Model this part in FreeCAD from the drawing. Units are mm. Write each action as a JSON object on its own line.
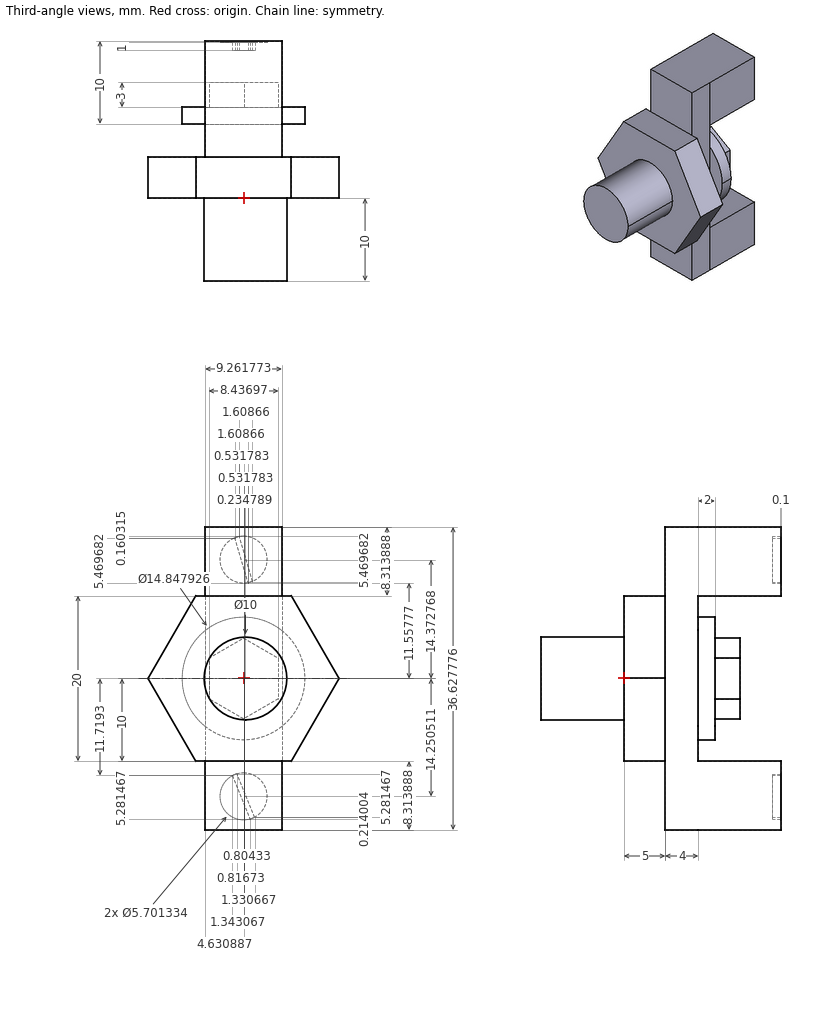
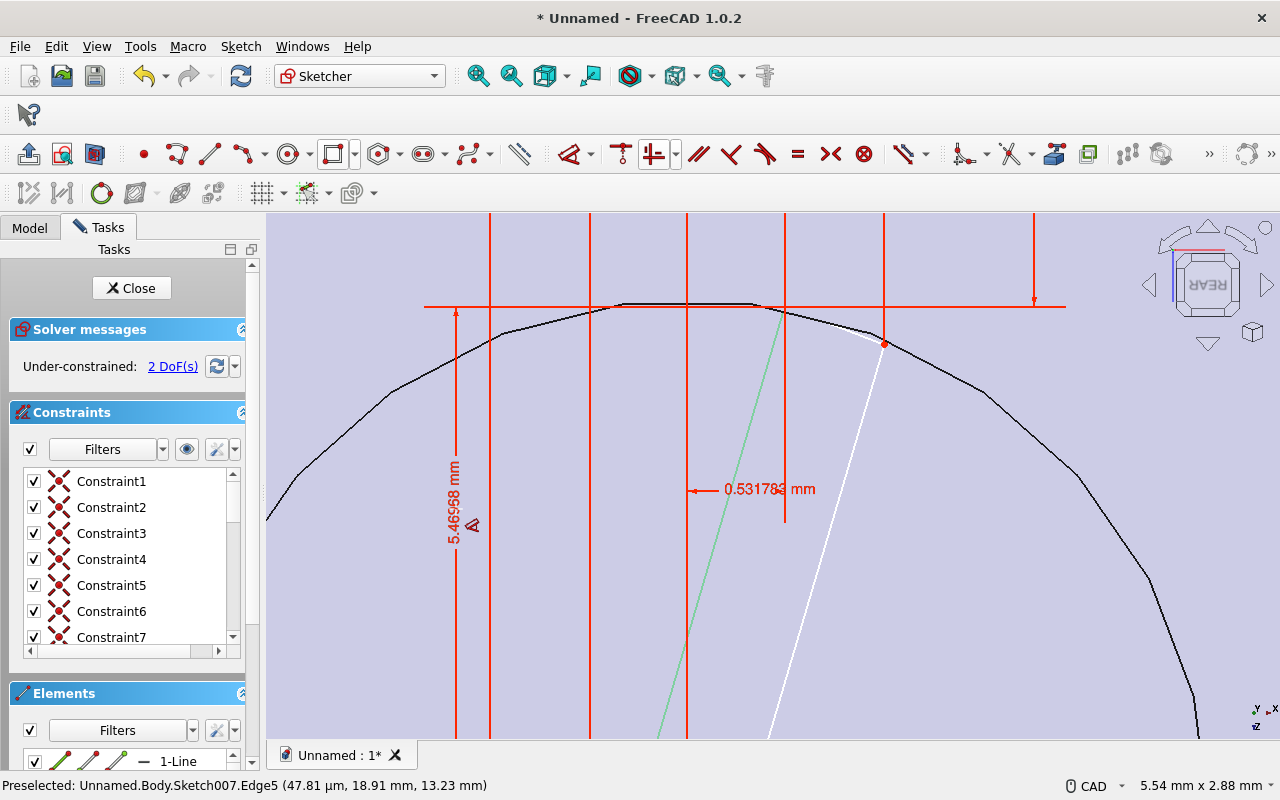
{"action": "scroll", "coordinate": [705, 595], "scroll_direction": "down", "scroll_amount": 15}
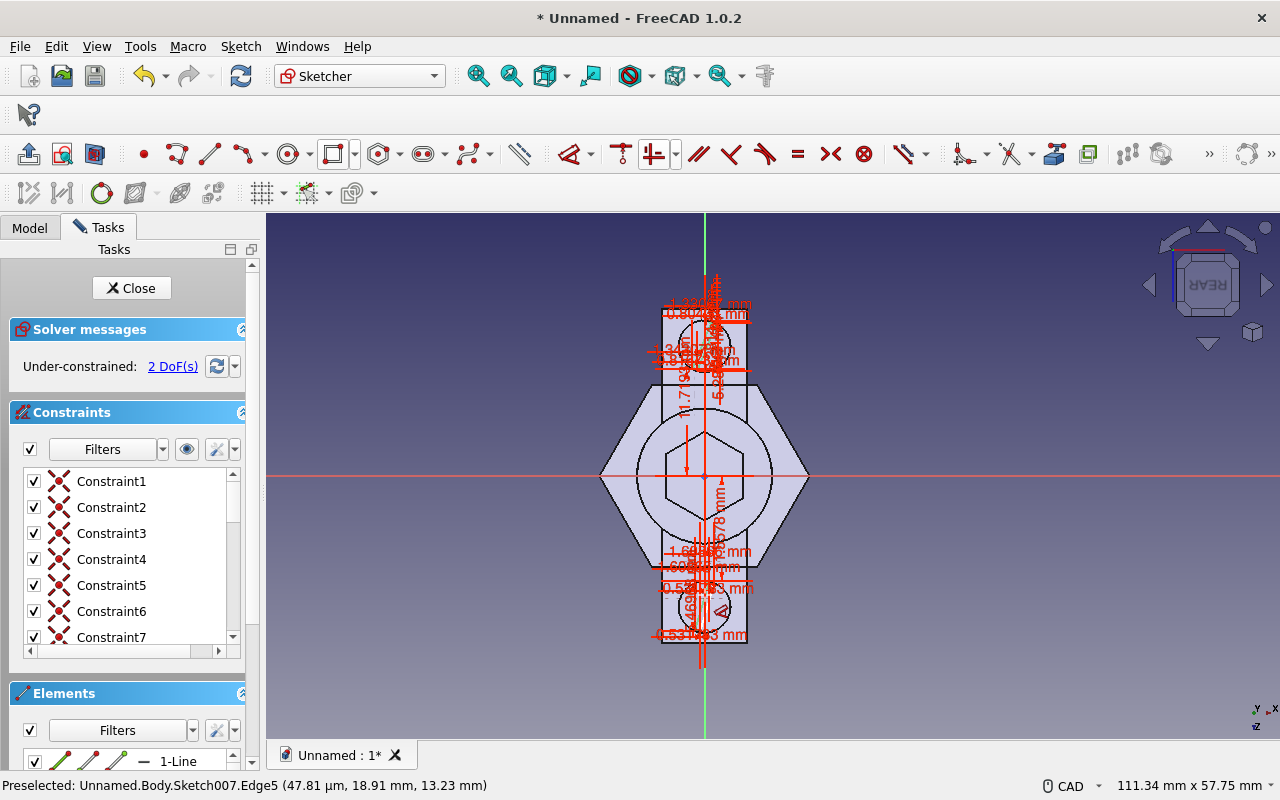
{"action": "scroll", "coordinate": [696, 632], "scroll_direction": "up", "scroll_amount": 17}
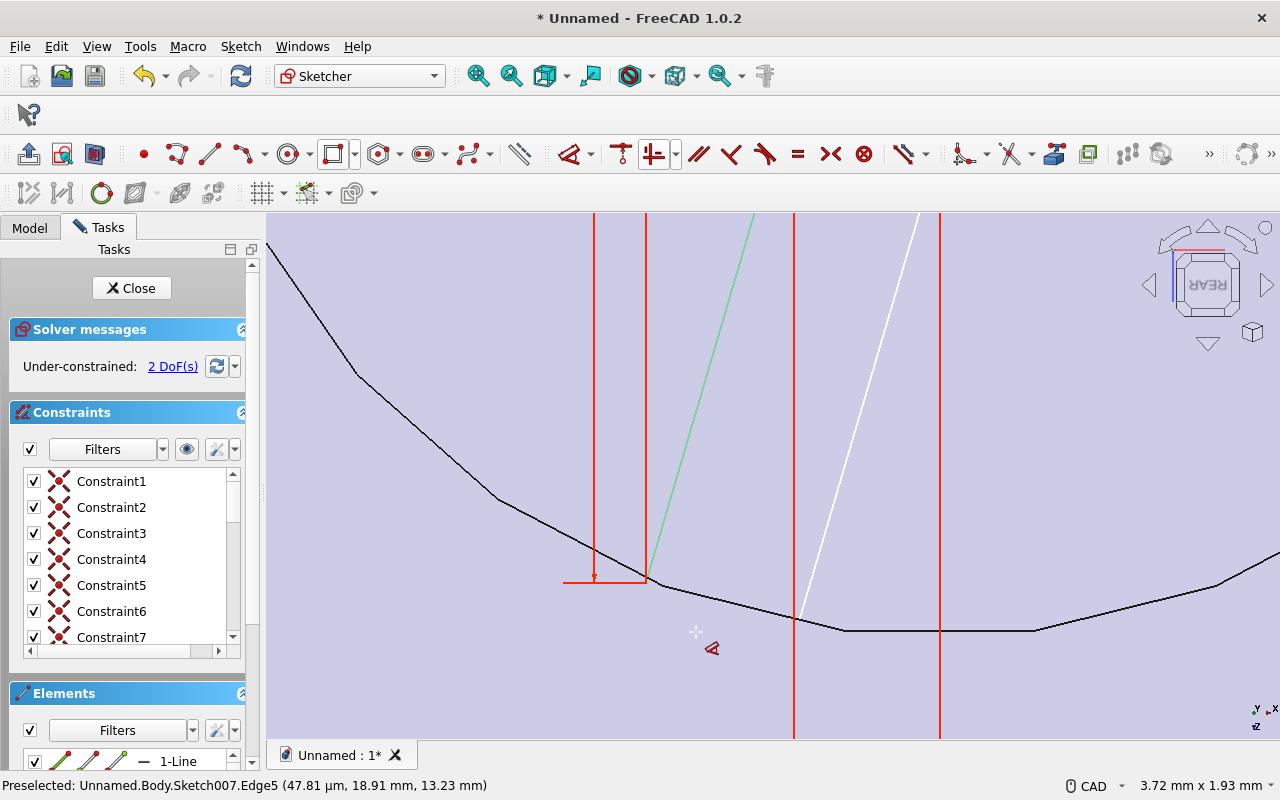
{"action": "left_click", "coordinate": [690, 599]}
{"action": "left_click", "coordinate": [612, 610]}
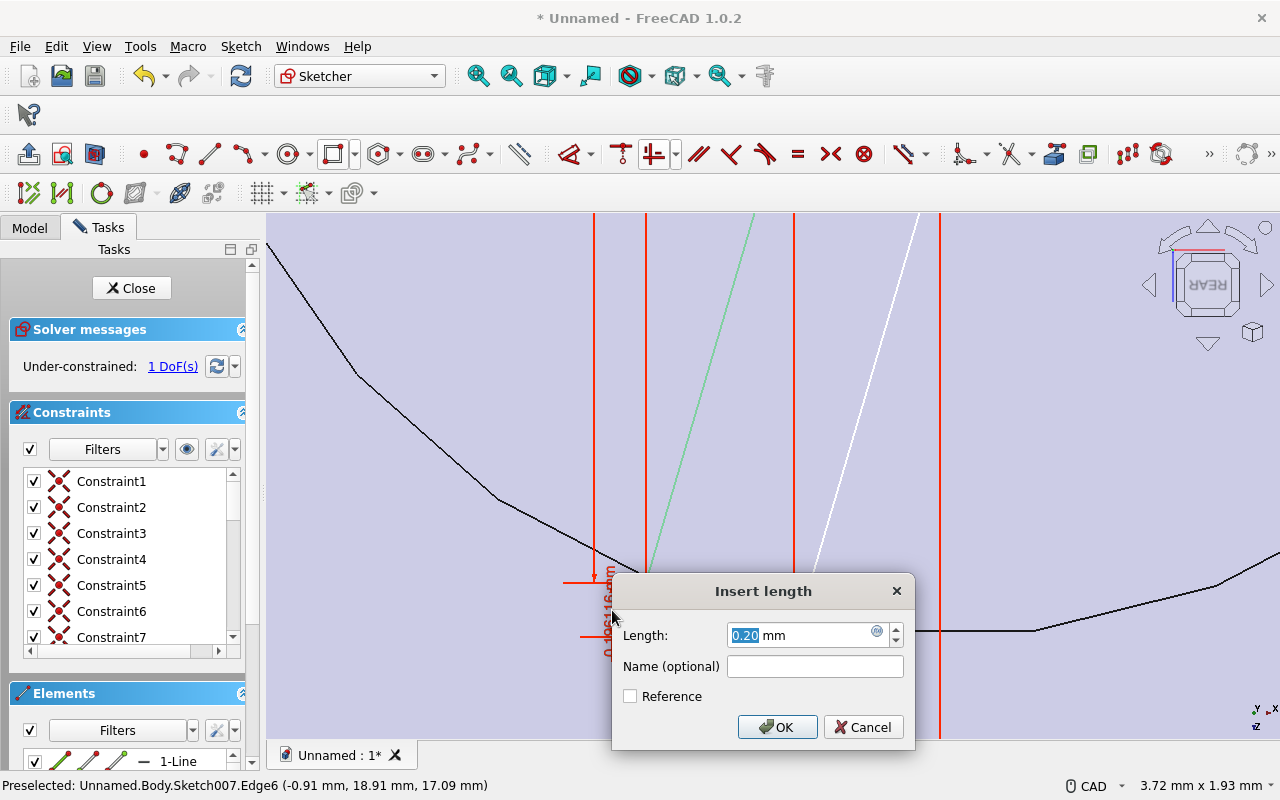
{"action": "type", "text": "0.160315"}
{"action": "key", "text": "Return"}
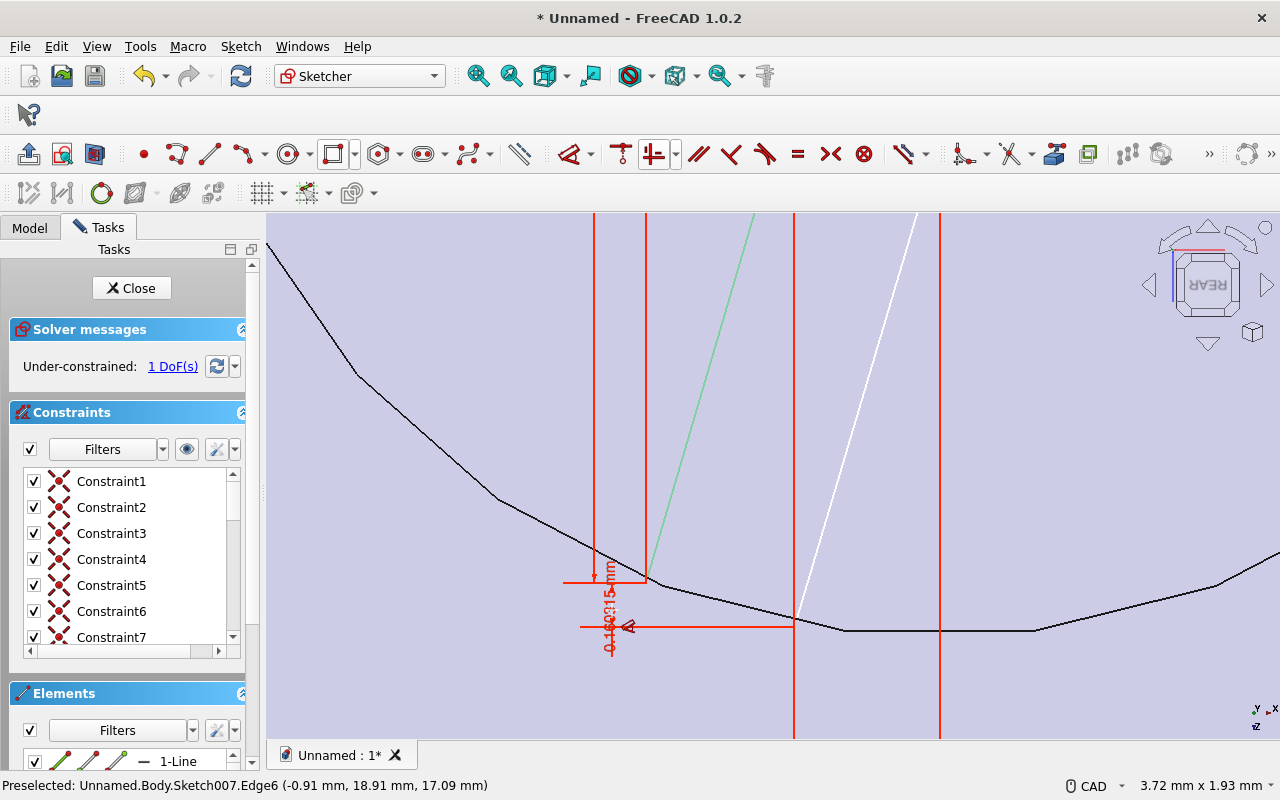
{"action": "scroll", "coordinate": [695, 668], "scroll_direction": "down", "scroll_amount": 16}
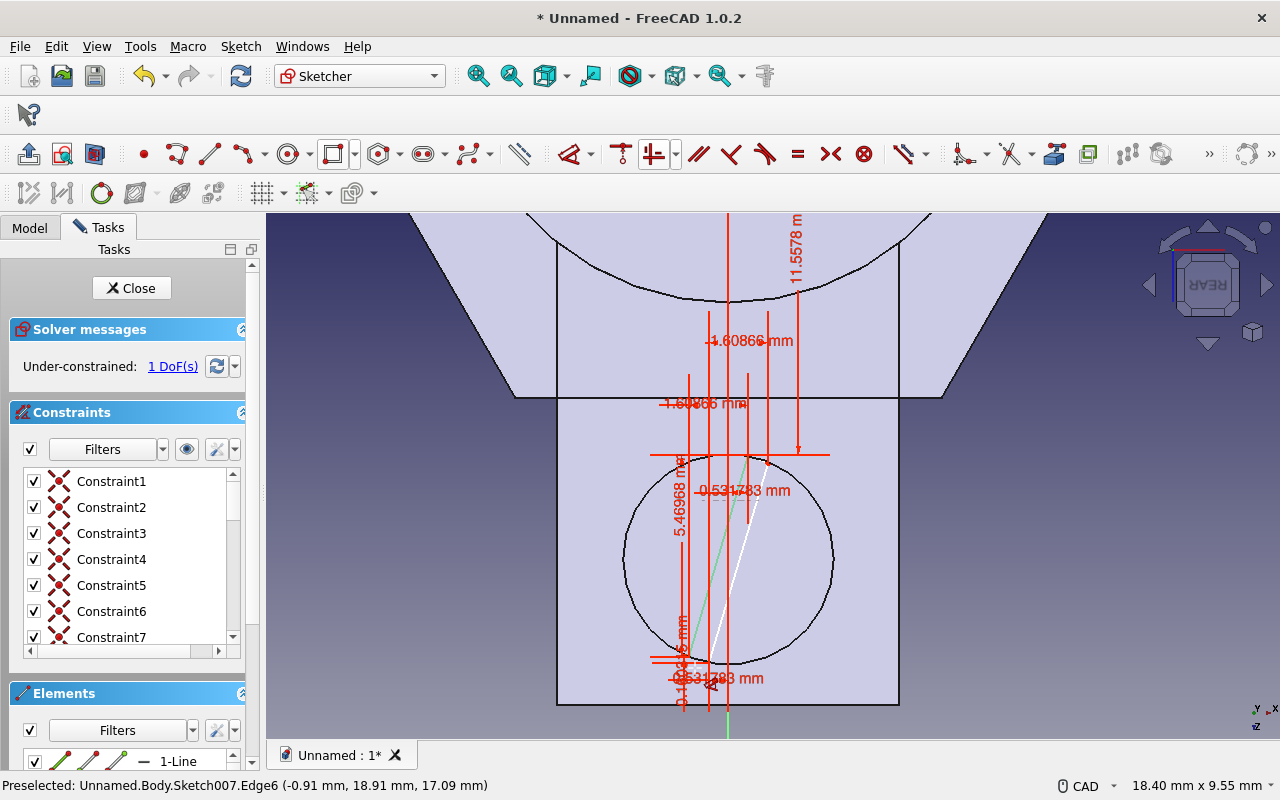
{"action": "scroll", "coordinate": [703, 655], "scroll_direction": "up", "scroll_amount": 9}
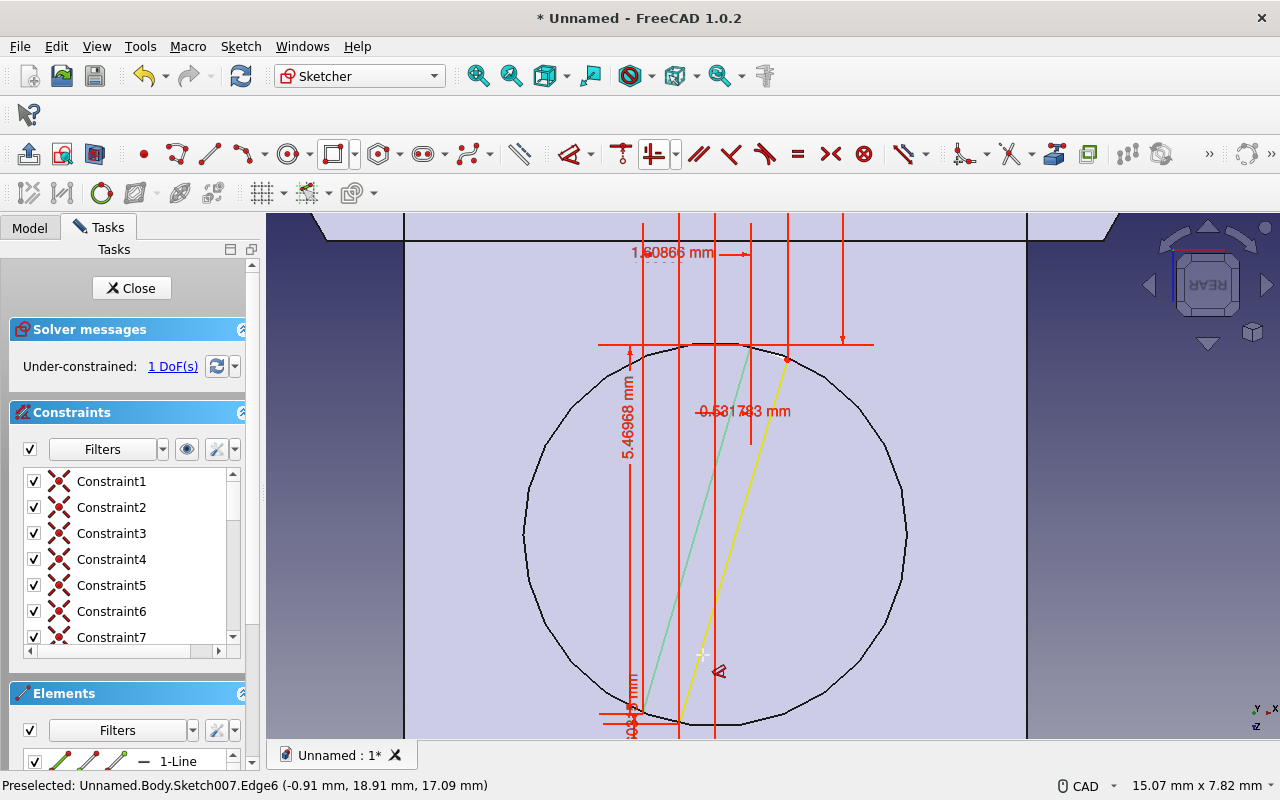
{"action": "left_click", "coordinate": [701, 651]}
{"action": "left_click", "coordinate": [822, 535]}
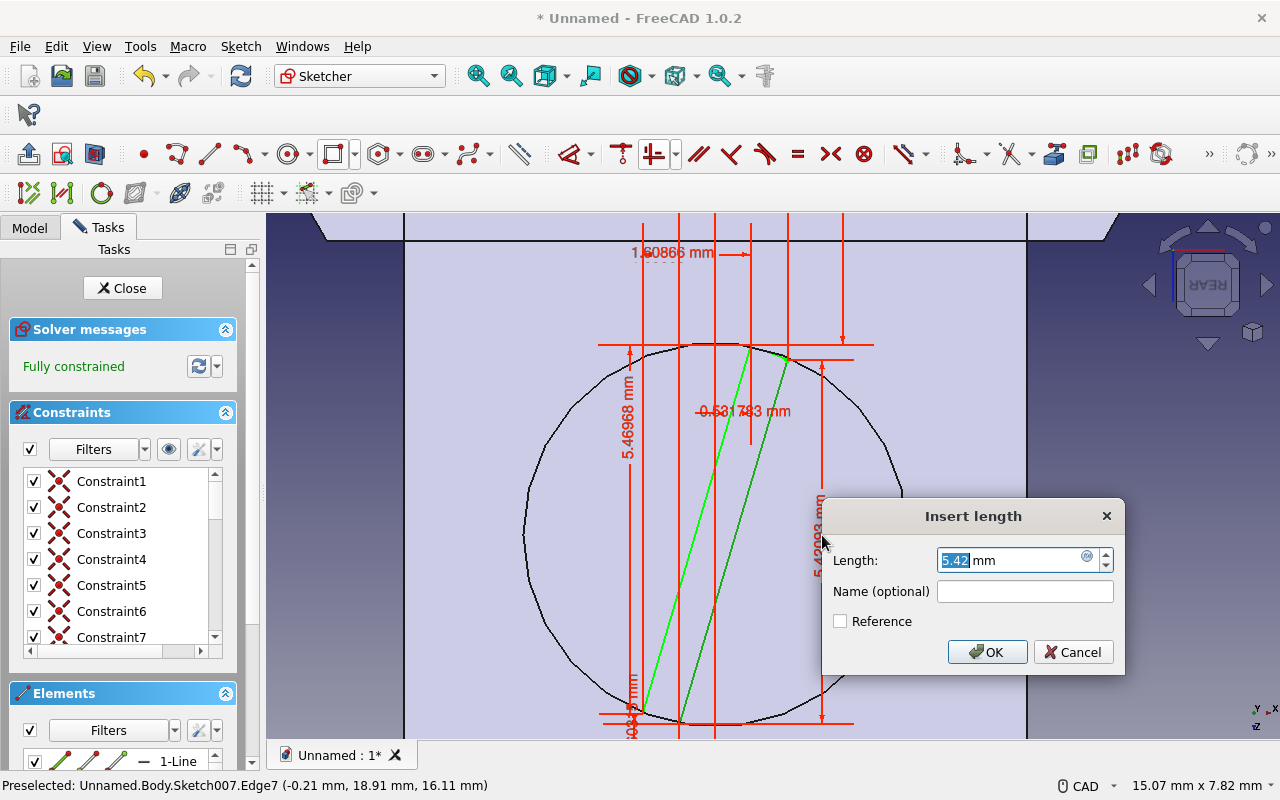
{"action": "type", "text": "5.469682"}
{"action": "key", "text": "Return"}
{"action": "key", "text": "Escape"}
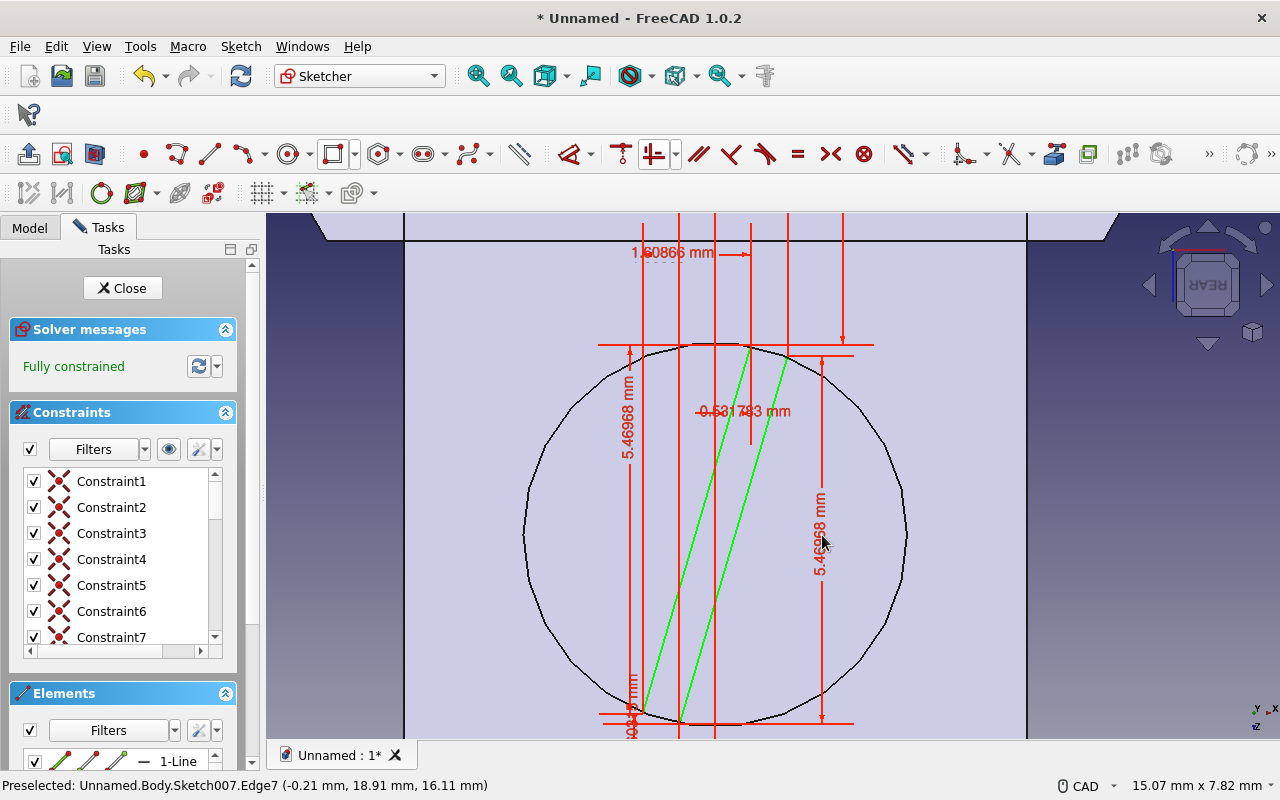
{"action": "left_click", "coordinate": [123, 288]}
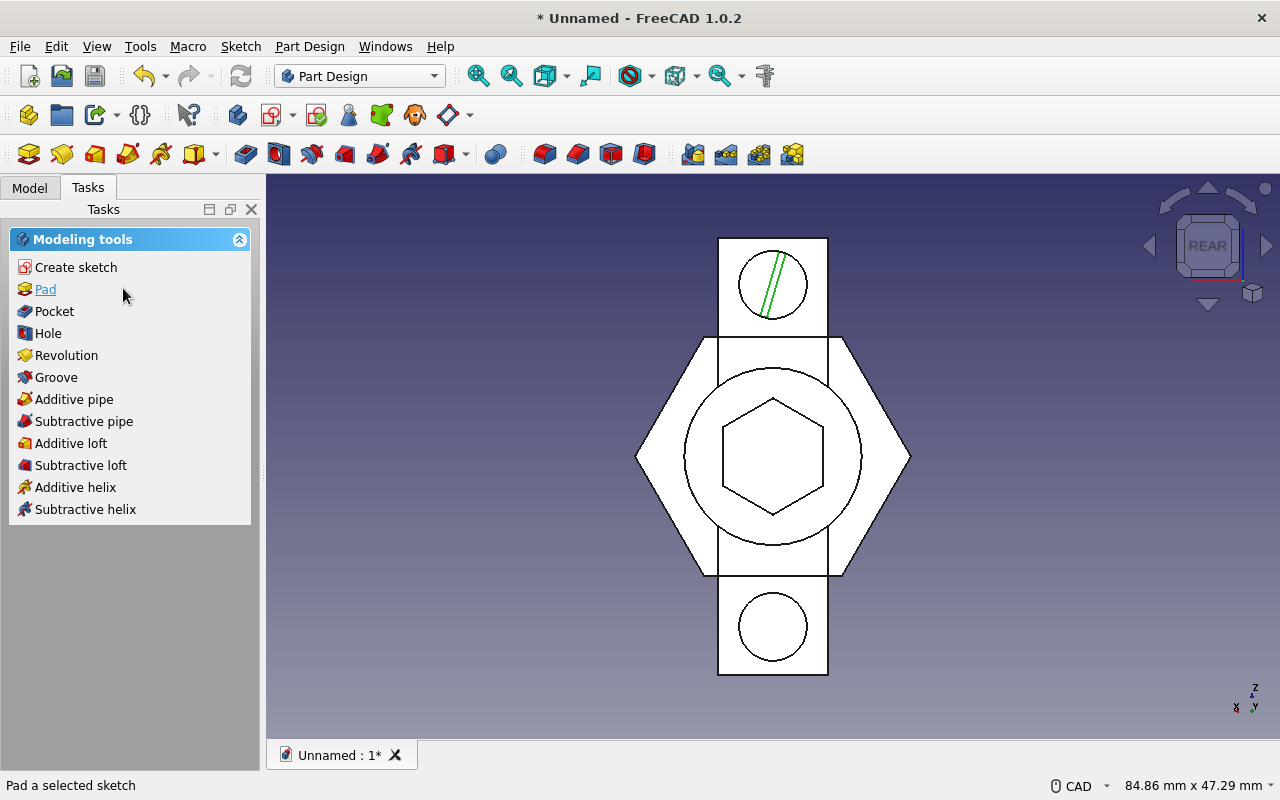
{"action": "left_click", "coordinate": [246, 154]}